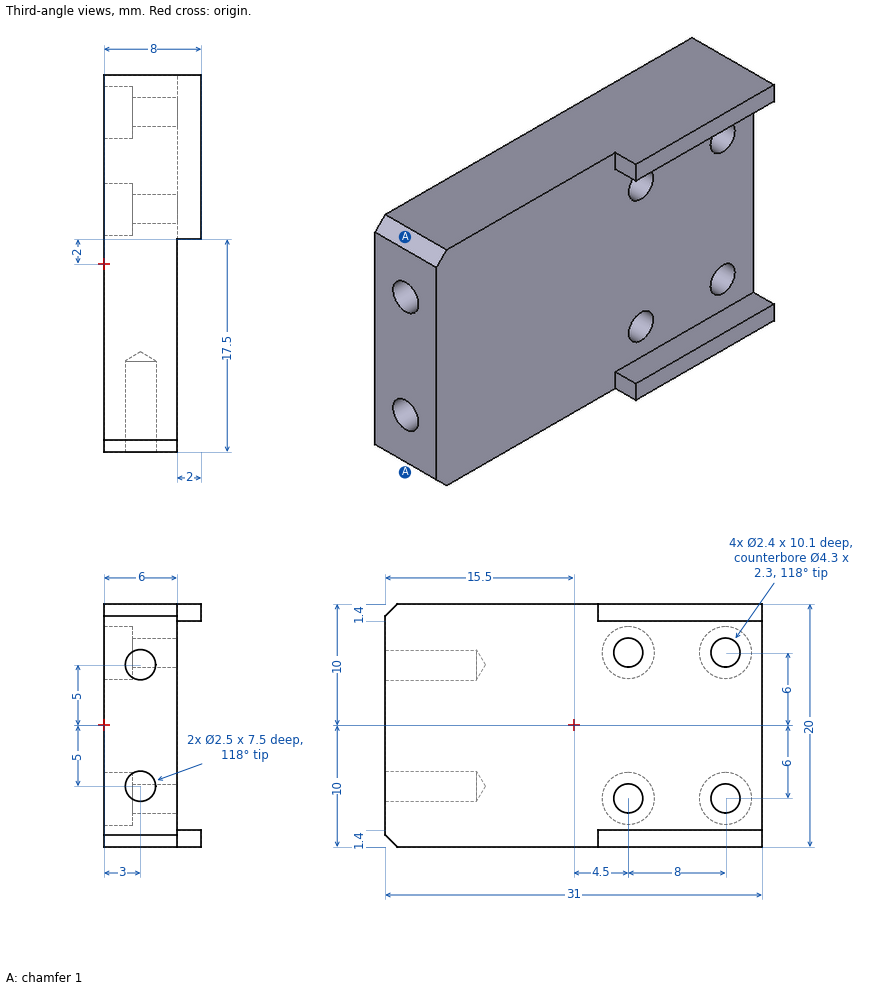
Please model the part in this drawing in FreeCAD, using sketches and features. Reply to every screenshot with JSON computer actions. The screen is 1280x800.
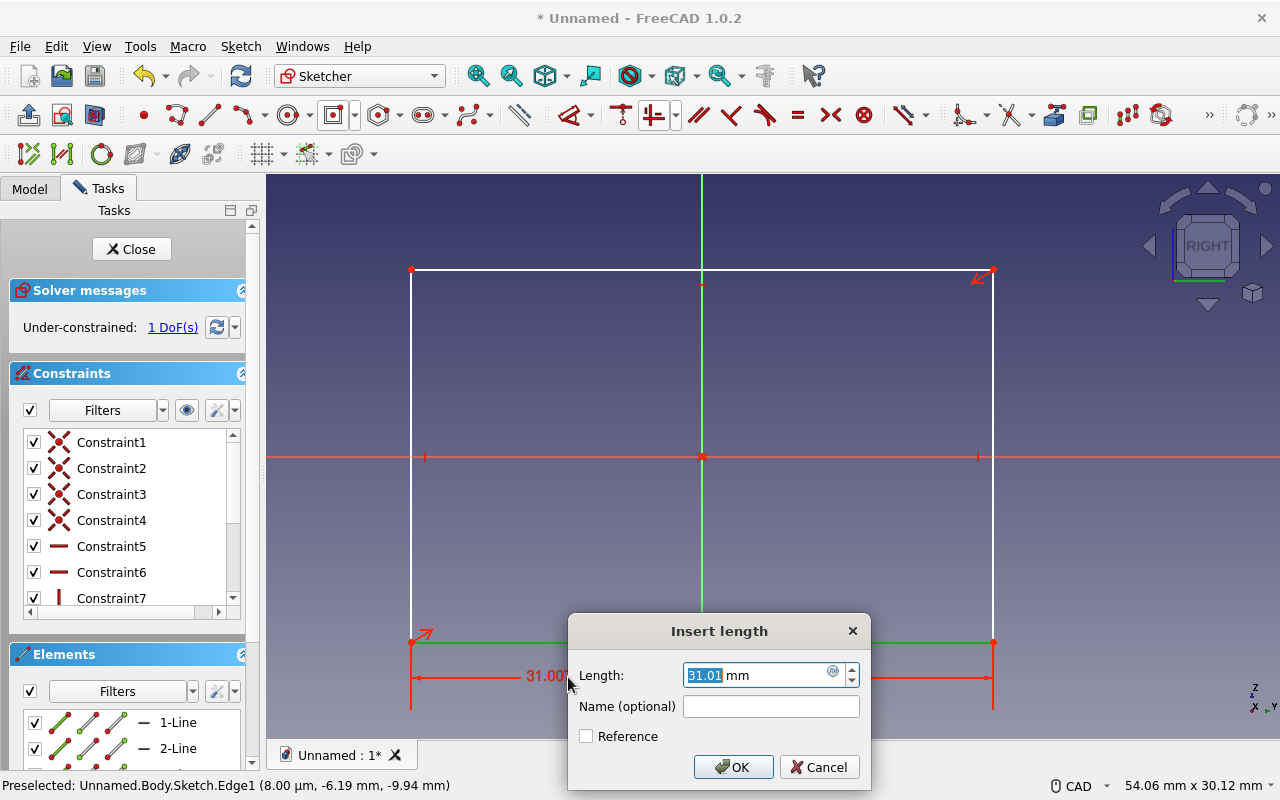
{"action": "type", "text": "31"}
{"action": "key", "text": "Return"}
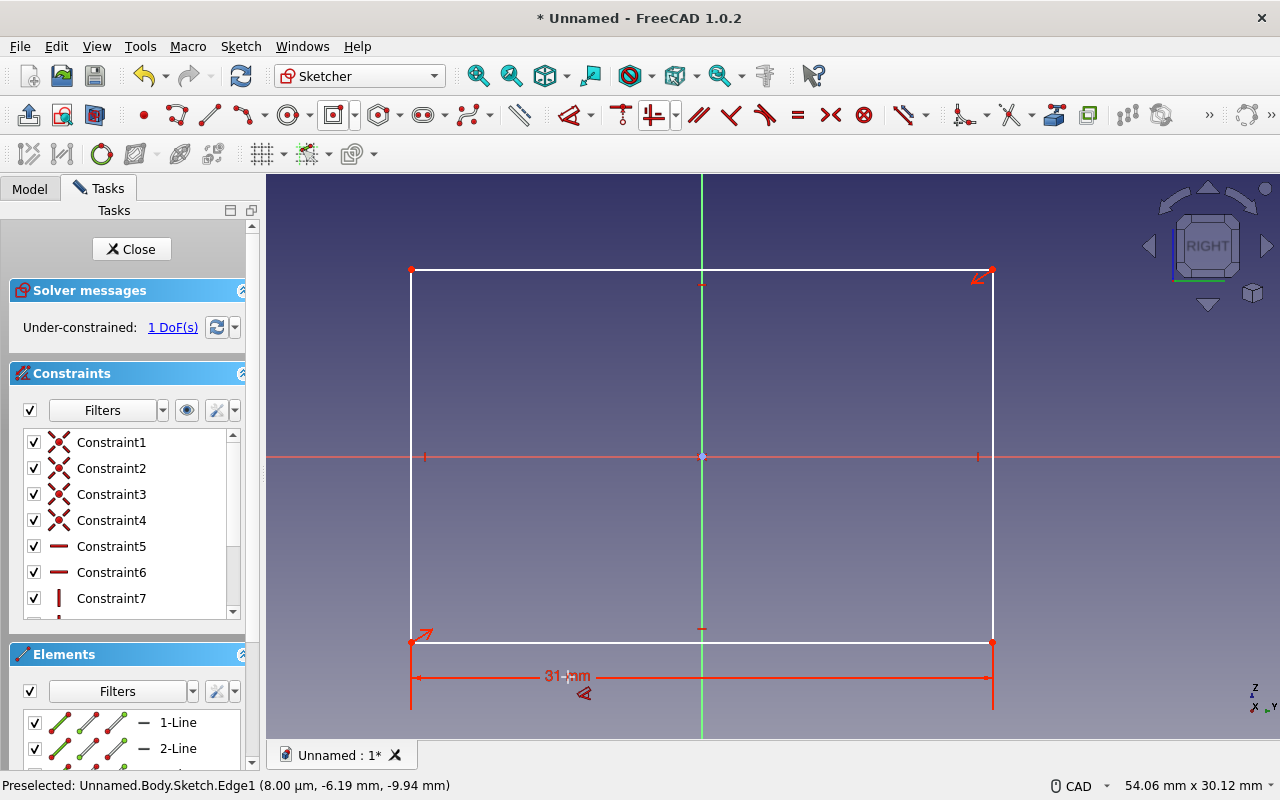
{"action": "left_click", "coordinate": [993, 531]}
{"action": "left_click", "coordinate": [1027, 371]}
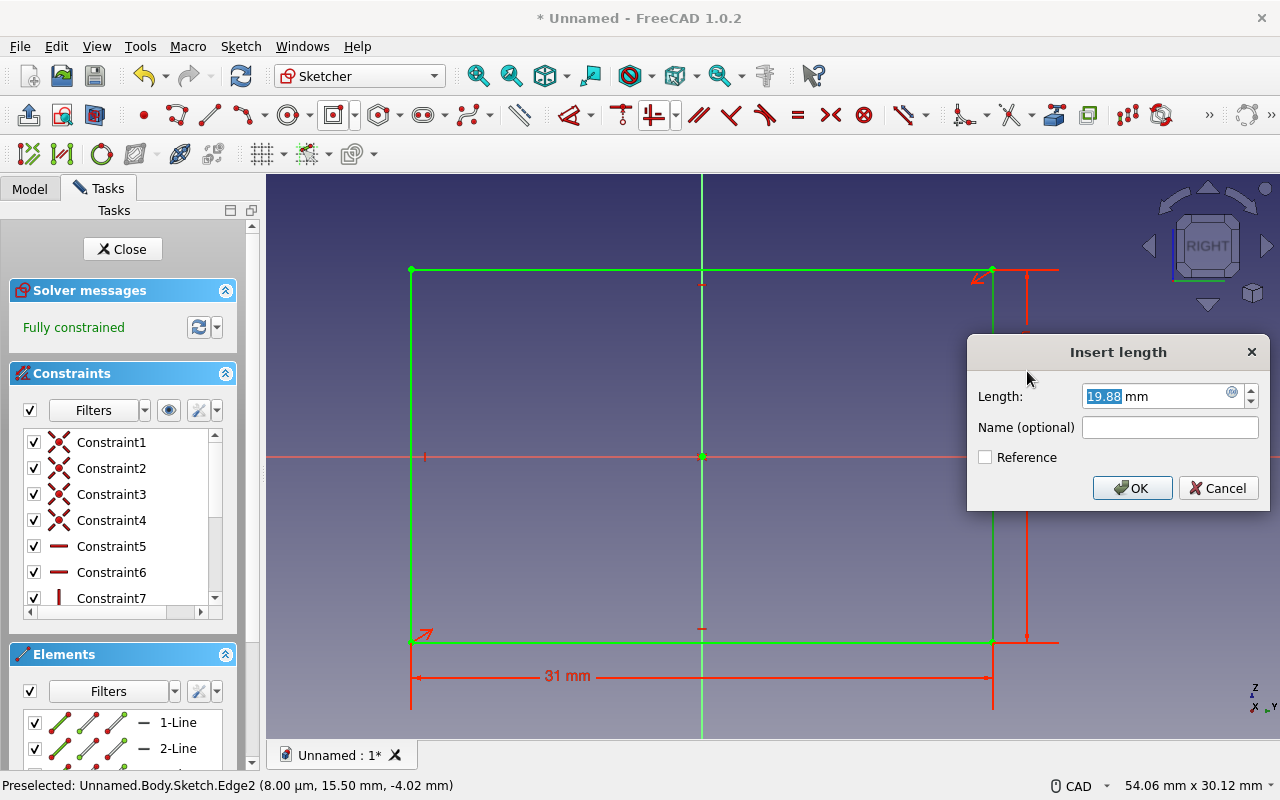
{"action": "type", "text": "20"}
{"action": "key", "text": "Return"}
{"action": "key", "text": "Escape"}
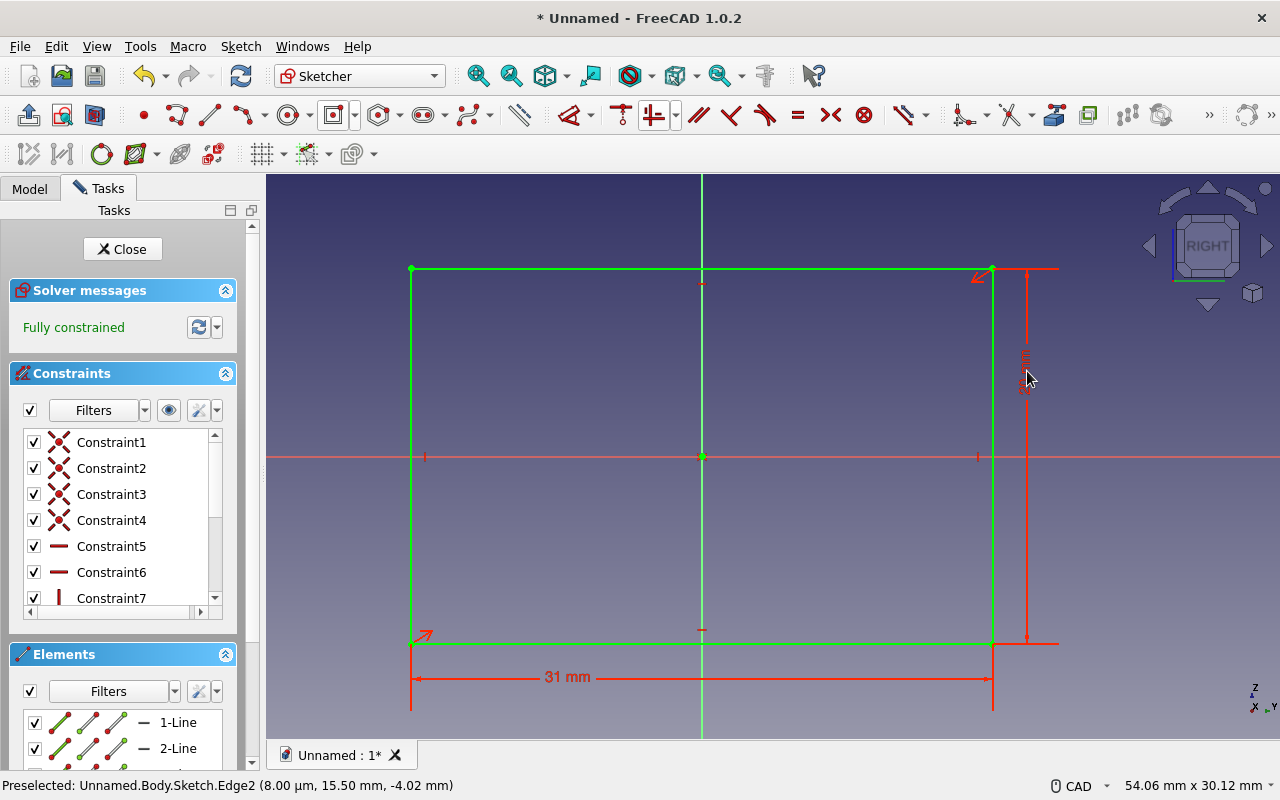
{"action": "left_click", "coordinate": [123, 249]}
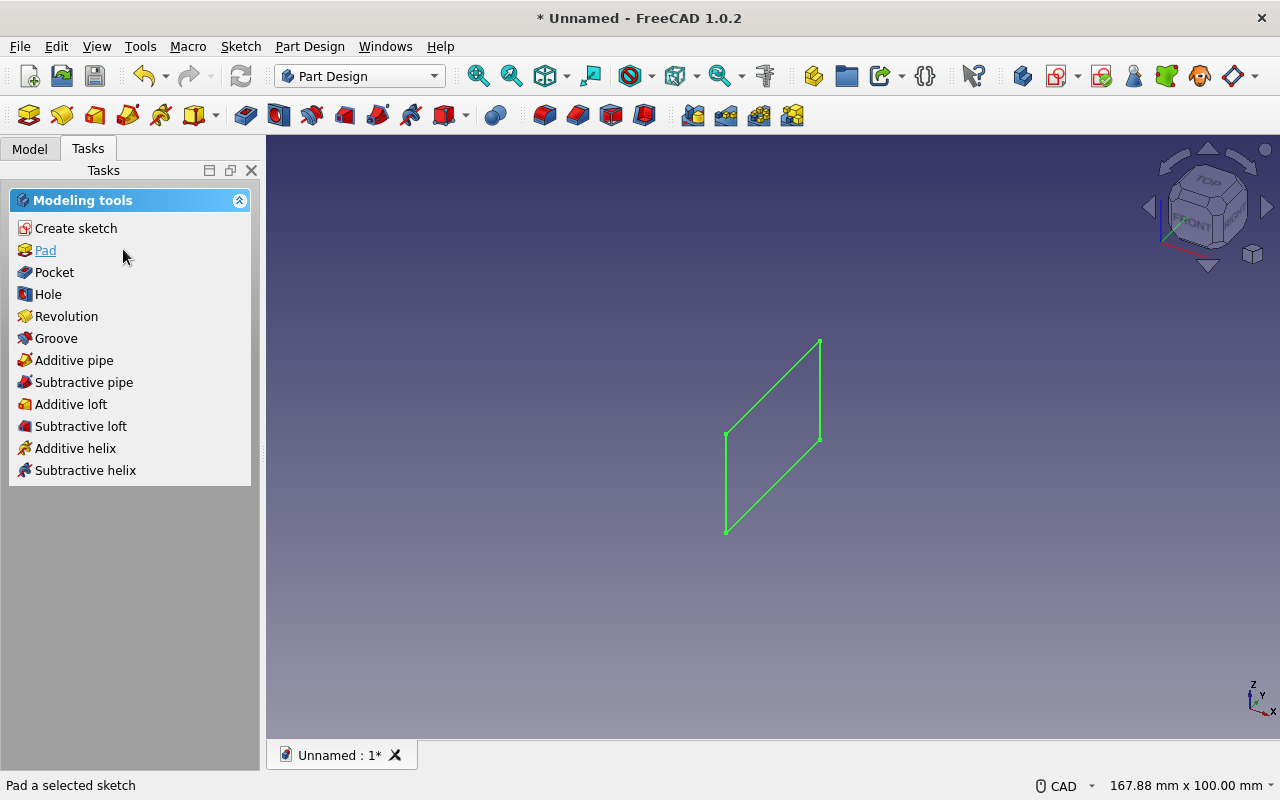
{"action": "left_click", "coordinate": [29, 116]}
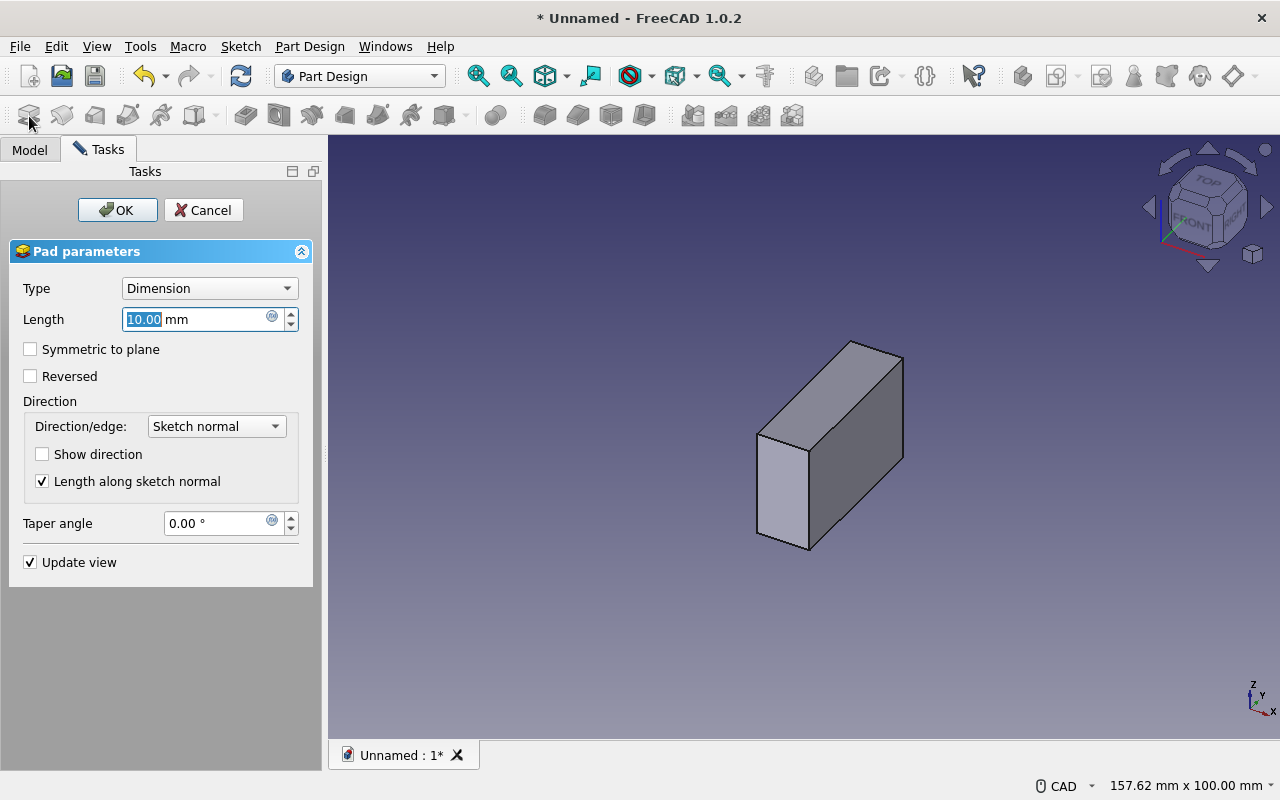
{"action": "type", "text": "6"}
{"action": "key", "text": "Tab"}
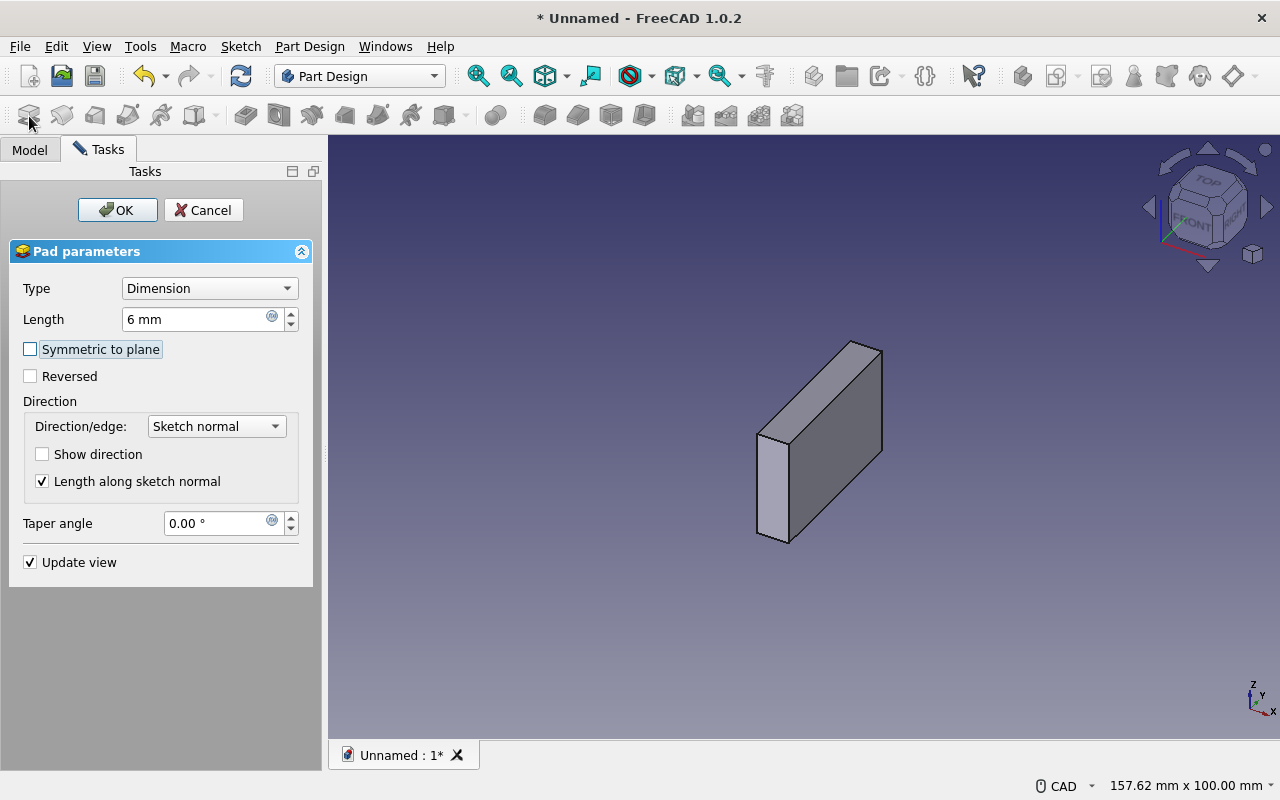
{"action": "left_click", "coordinate": [118, 210]}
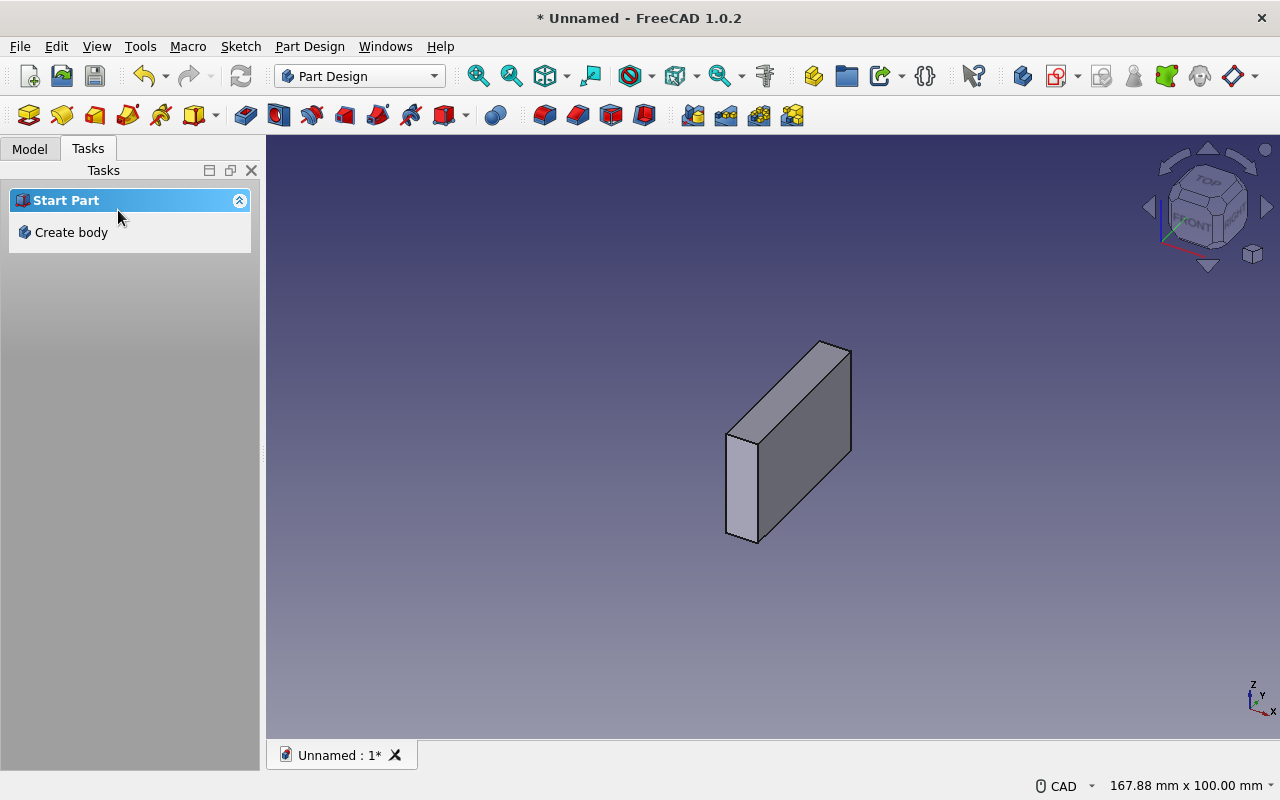
{"action": "key", "text": "v f"}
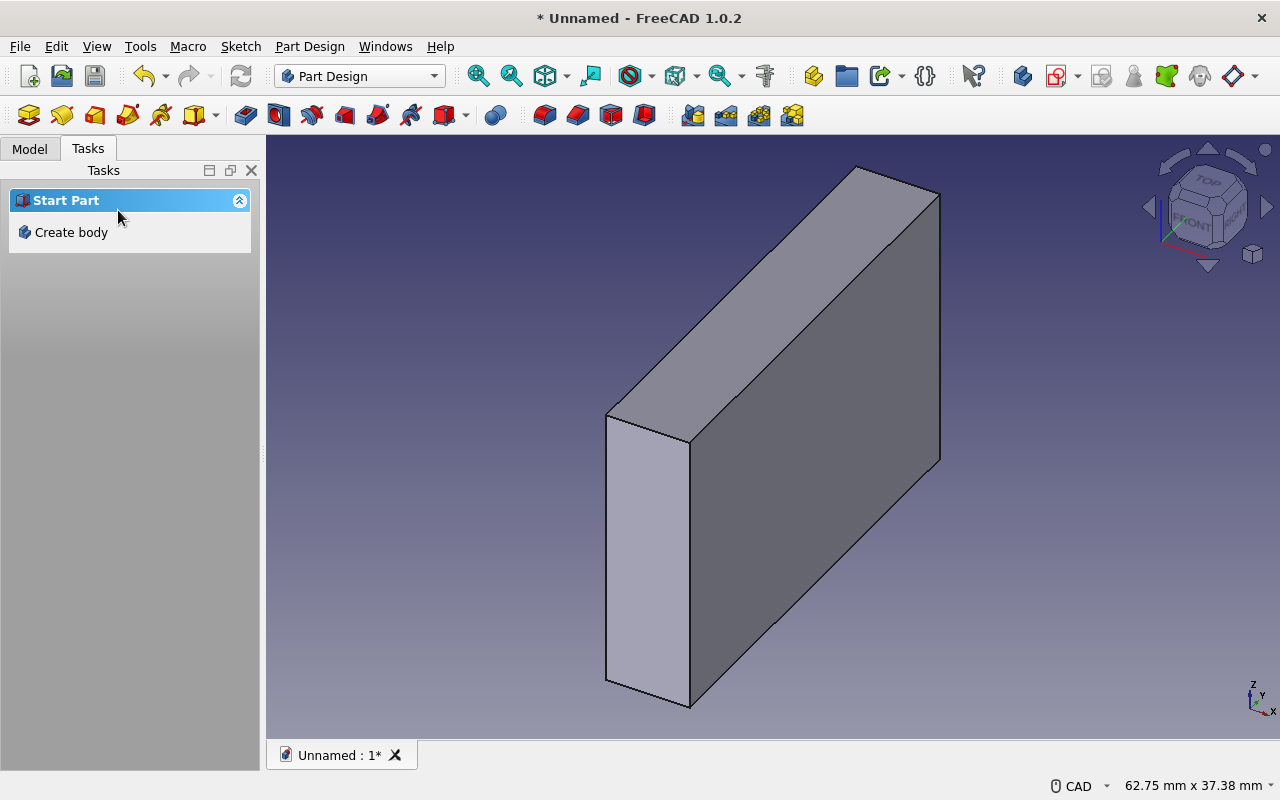
{"action": "left_click", "coordinate": [815, 450]}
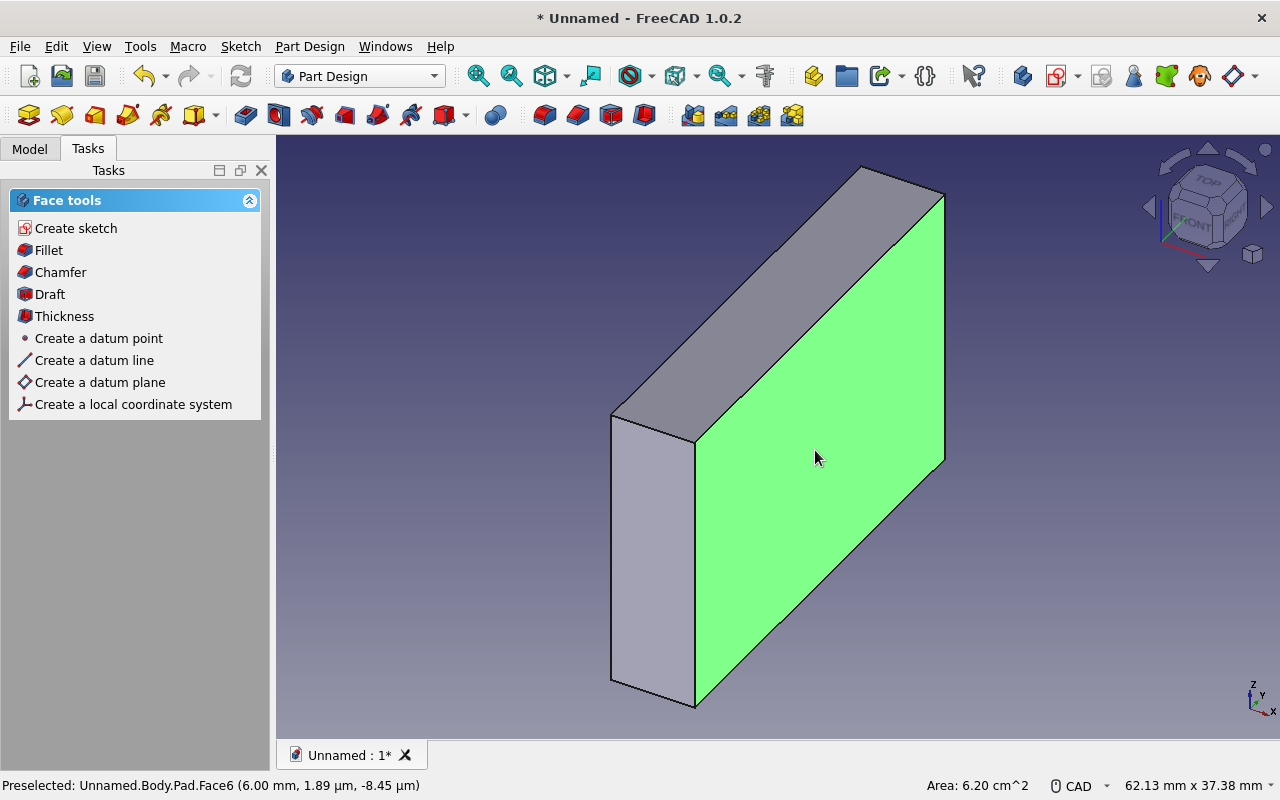
{"action": "left_click", "coordinate": [1056, 76]}